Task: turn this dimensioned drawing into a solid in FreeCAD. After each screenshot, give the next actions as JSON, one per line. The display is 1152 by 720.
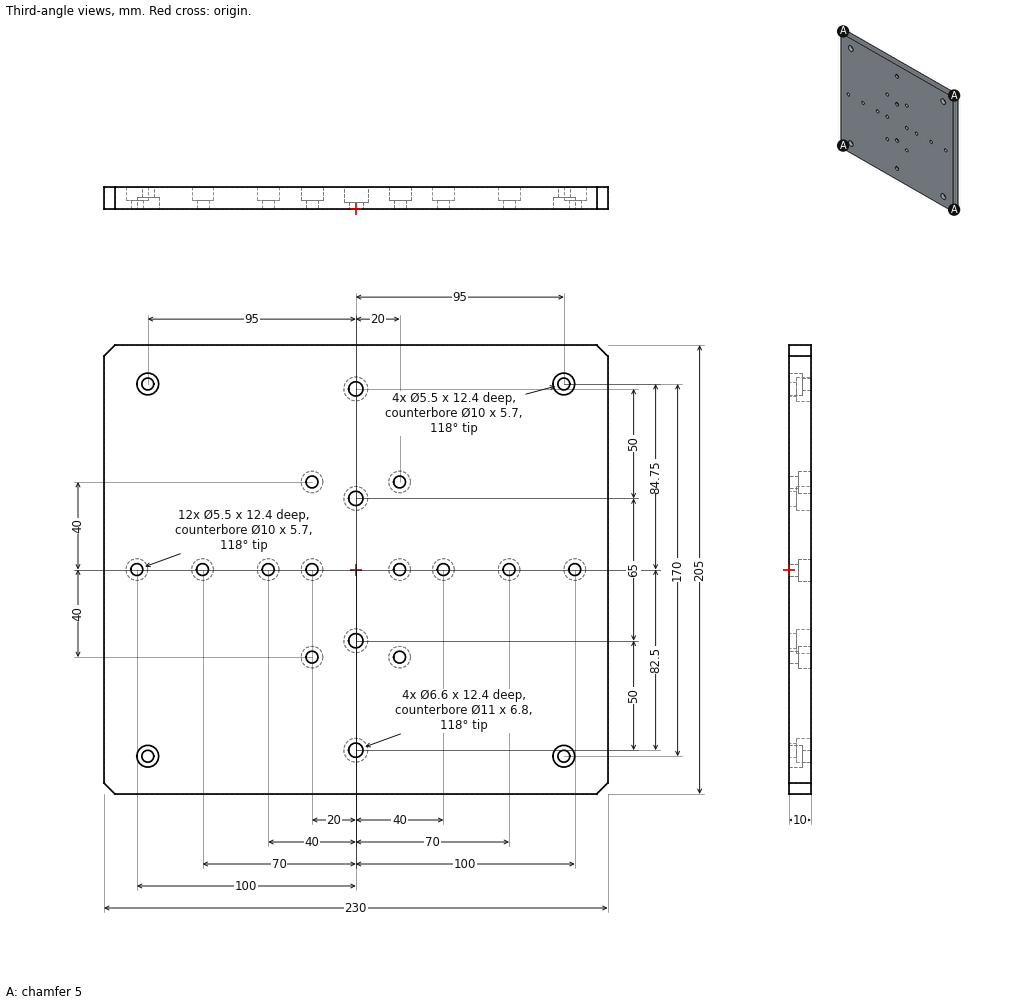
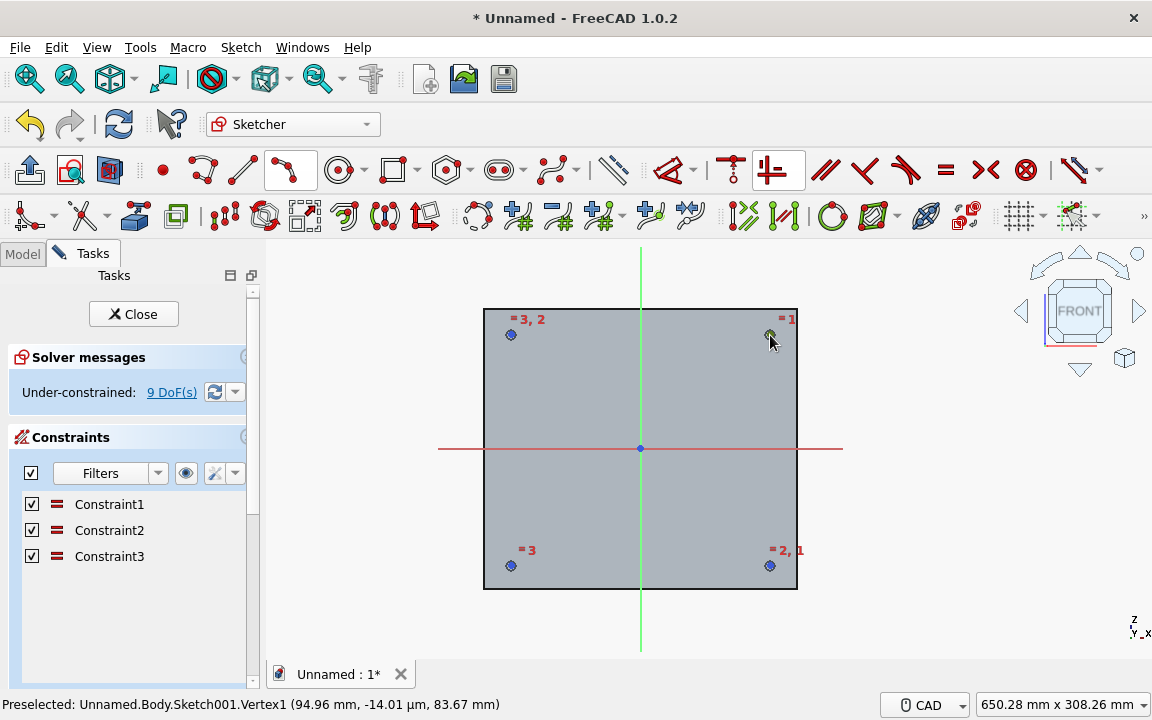
{"action": "left_click", "coordinate": [770, 566]}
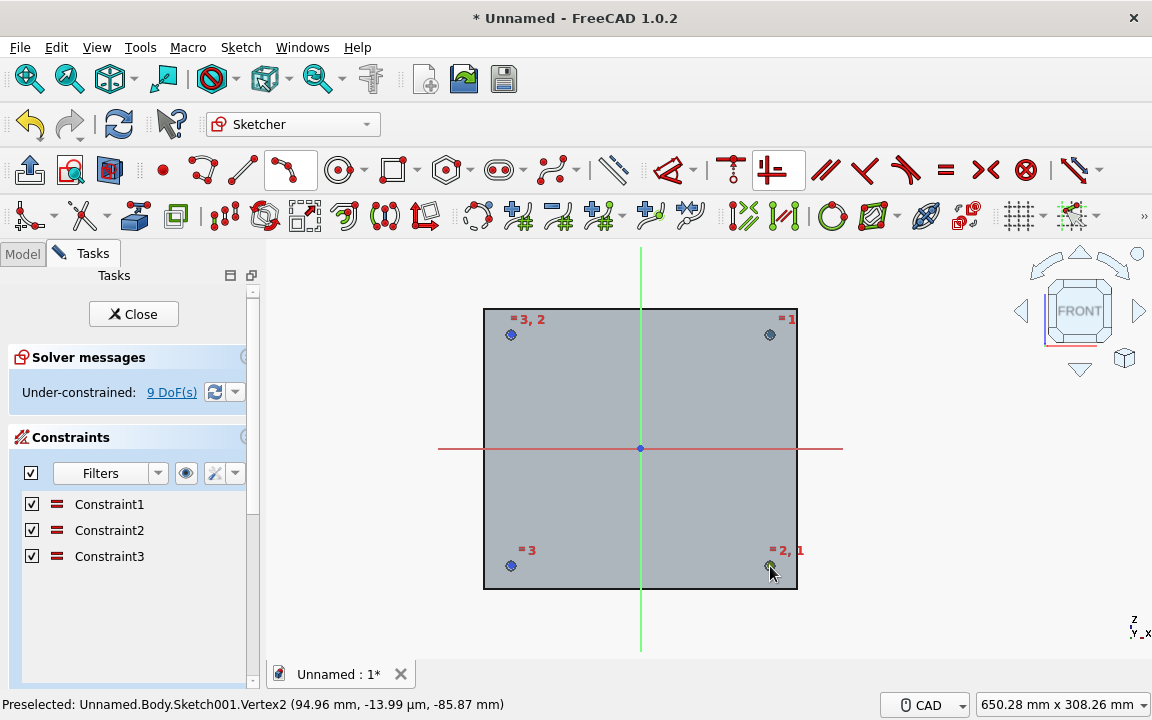
{"action": "left_click", "coordinate": [800, 170]}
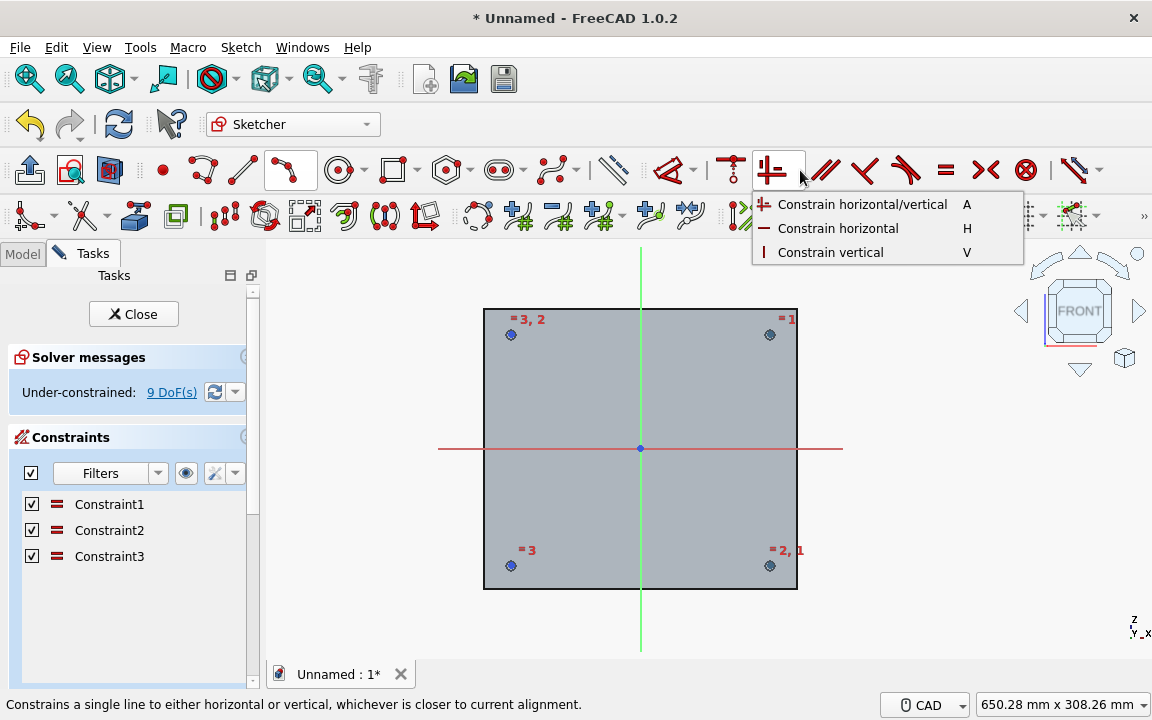
{"action": "left_click", "coordinate": [888, 252]}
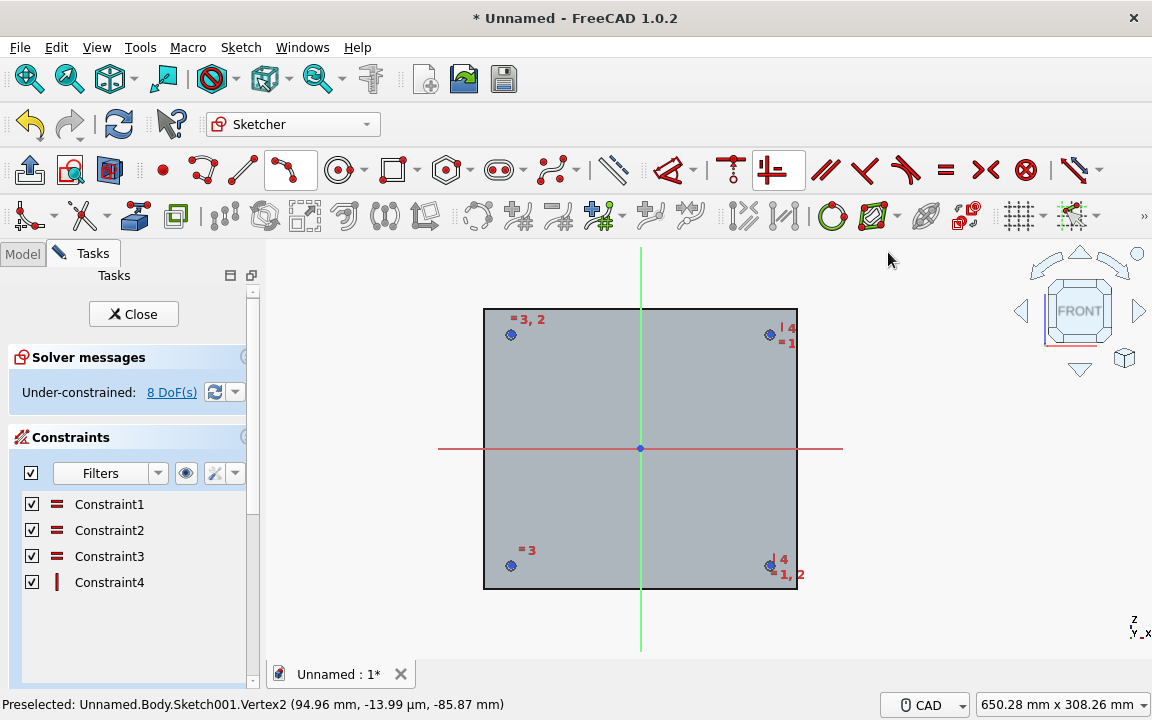
{"action": "left_click", "coordinate": [770, 335]}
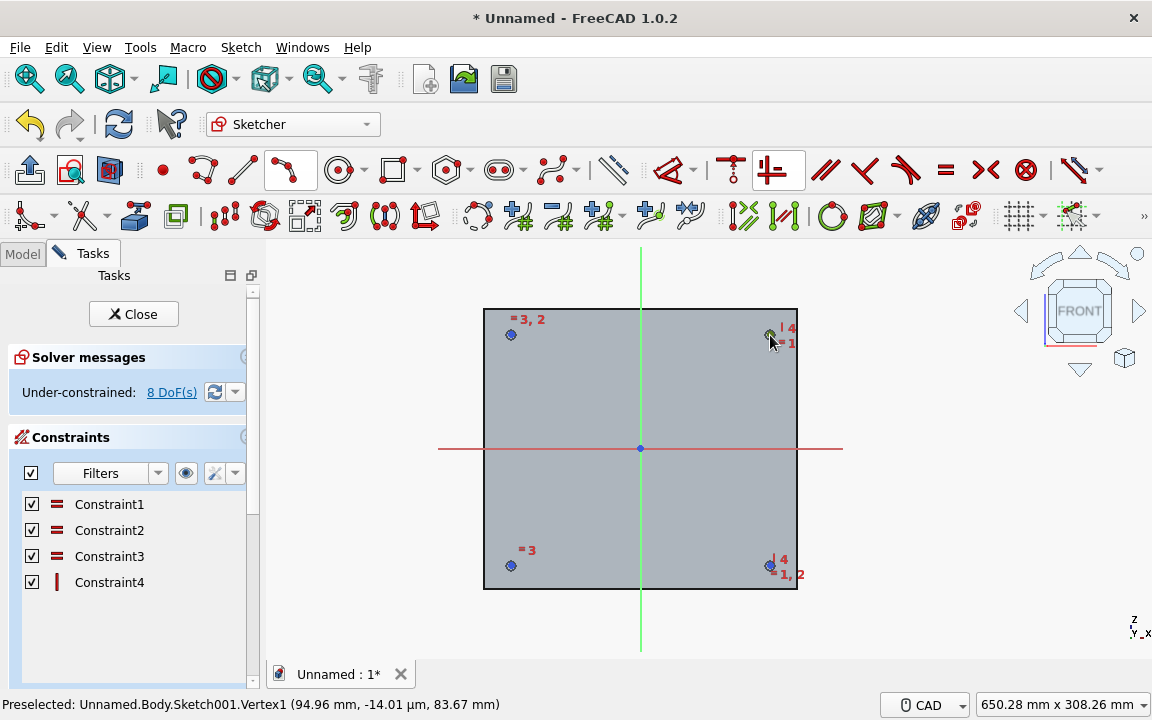
{"action": "left_click", "coordinate": [511, 335]}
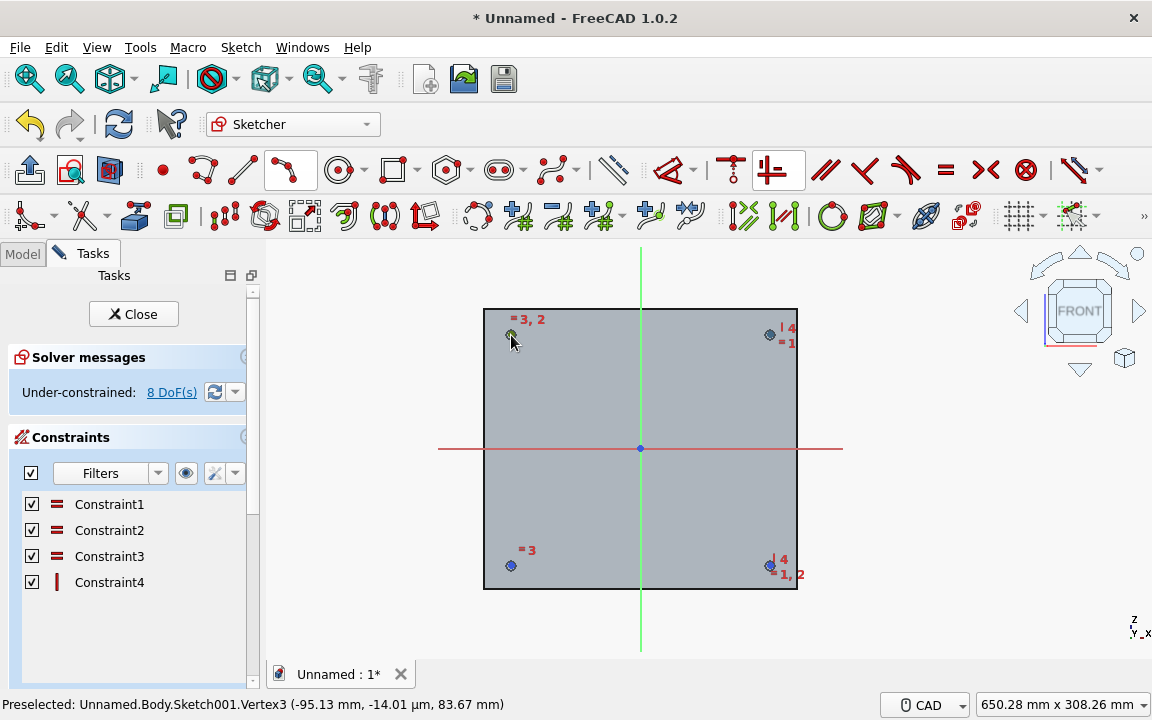
{"action": "left_click", "coordinate": [800, 170]}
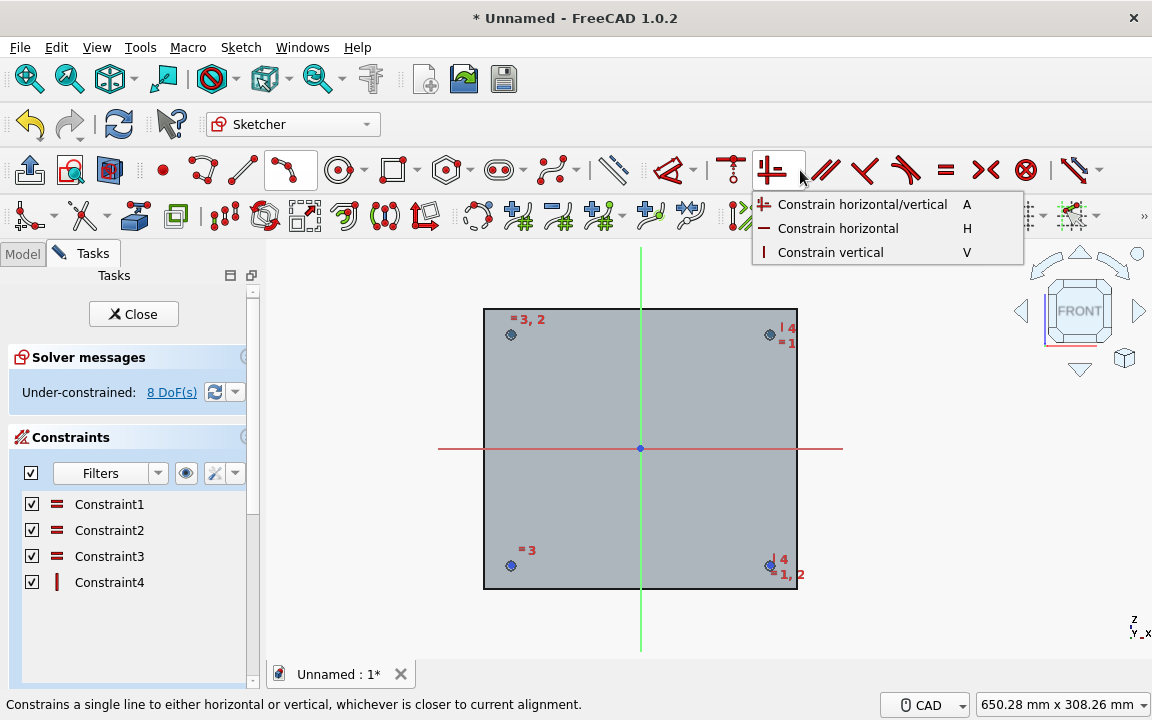
{"action": "left_click", "coordinate": [888, 228]}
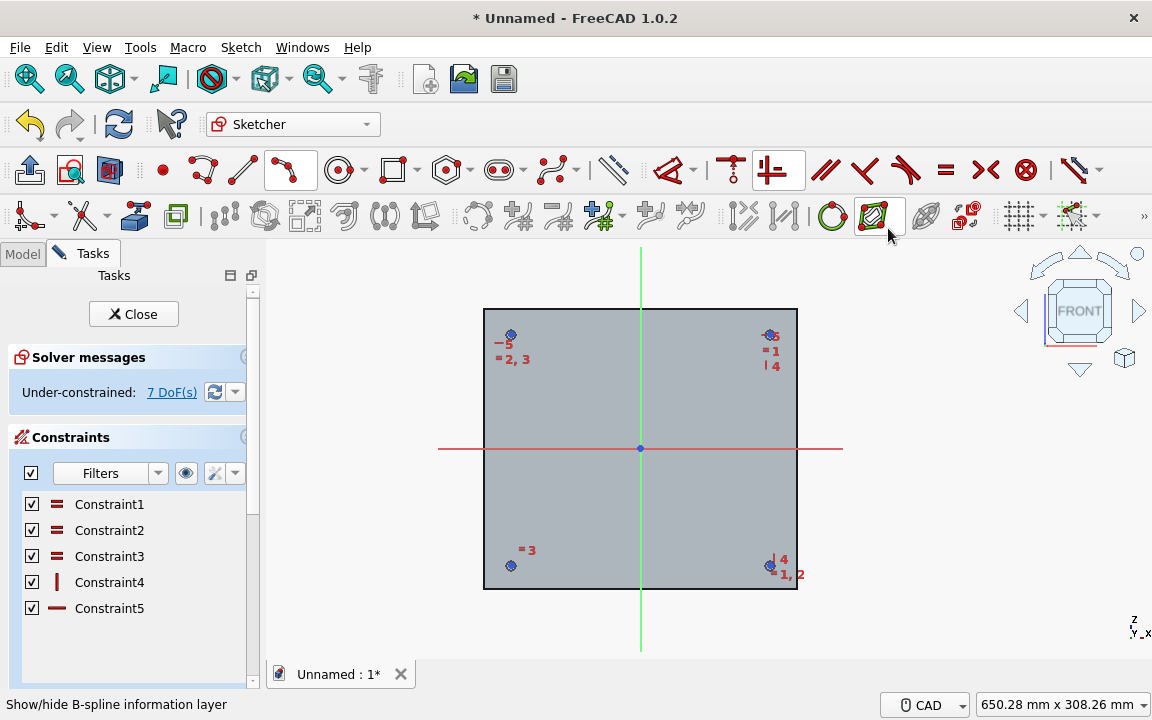
{"action": "left_click", "coordinate": [511, 335]}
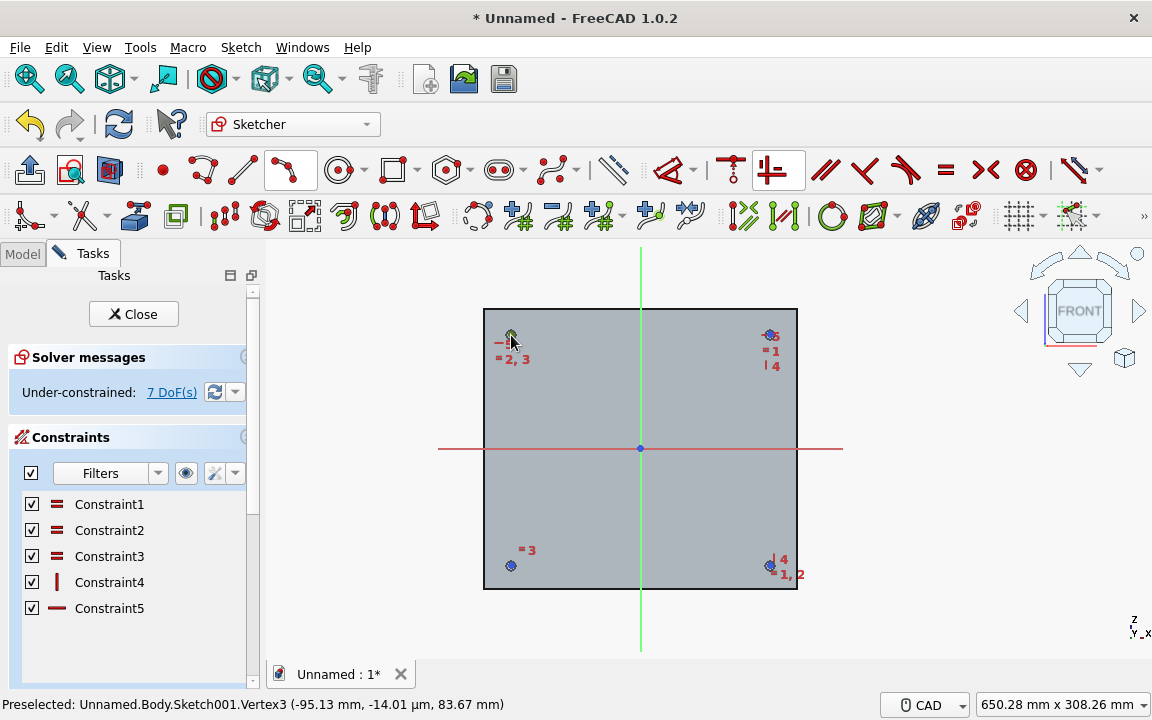
{"action": "left_click", "coordinate": [511, 566]}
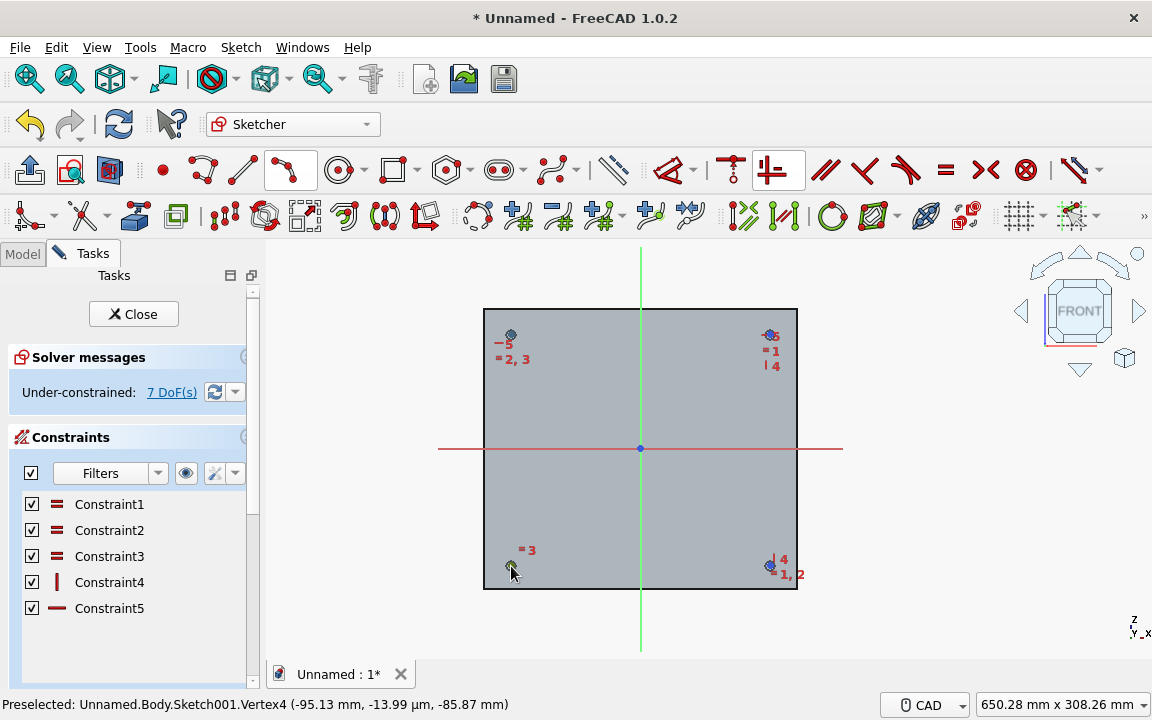
{"action": "key", "text": "v"}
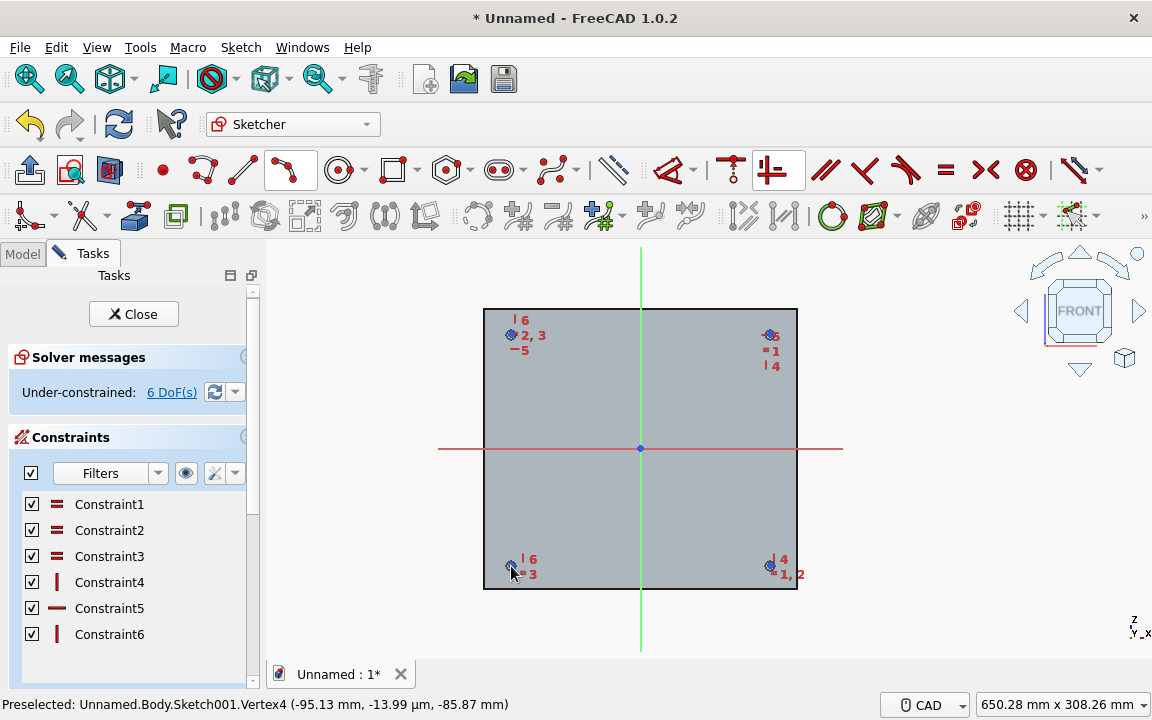
{"action": "left_click", "coordinate": [768, 568]}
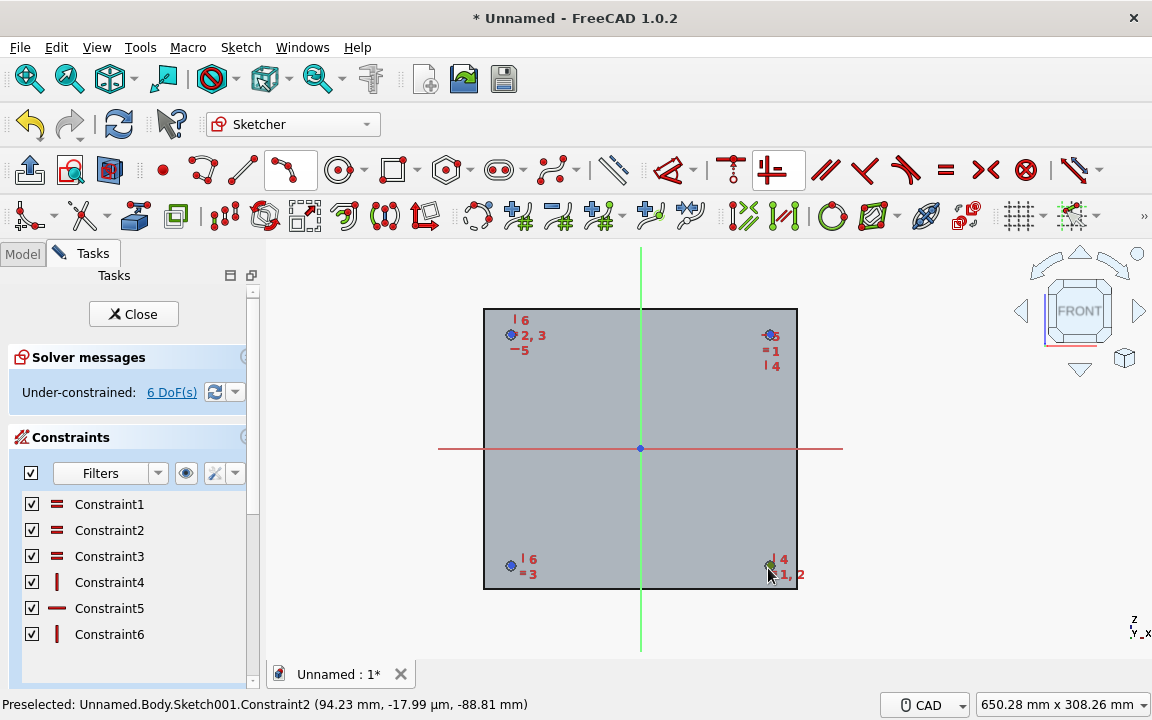
{"action": "left_click", "coordinate": [511, 566]}